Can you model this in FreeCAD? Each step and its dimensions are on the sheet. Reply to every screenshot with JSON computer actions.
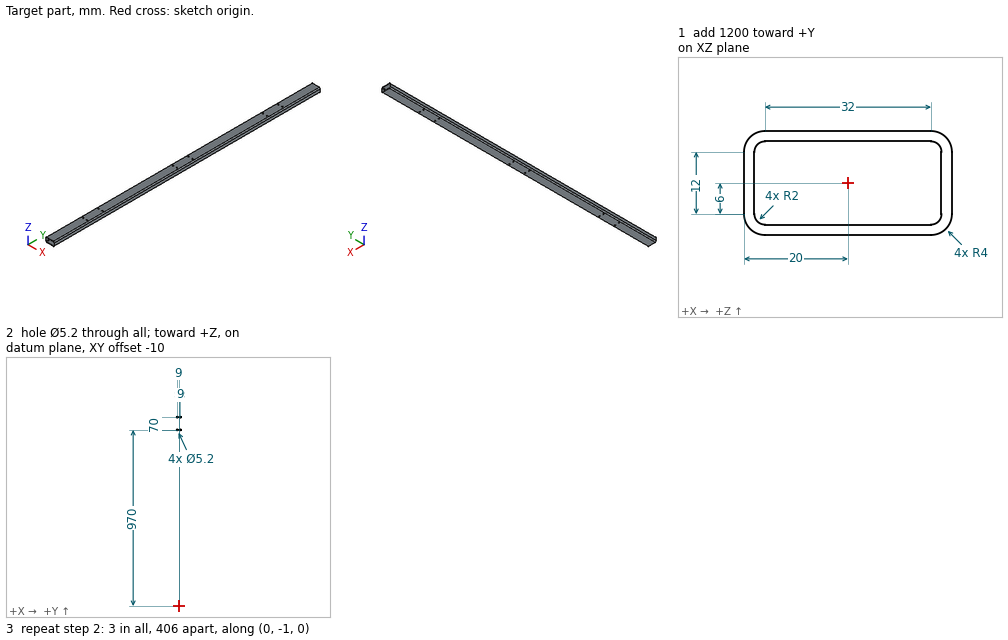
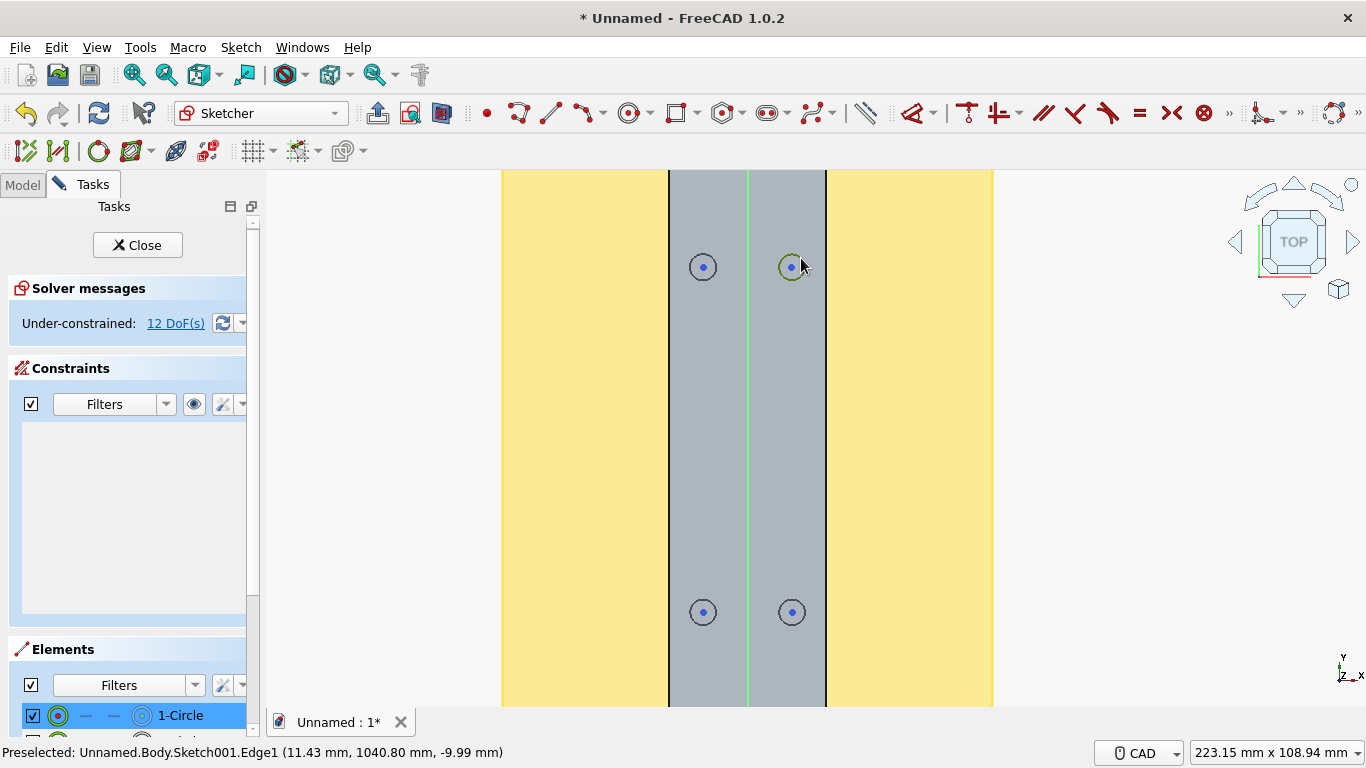
{"action": "left_click", "coordinate": [712, 258]}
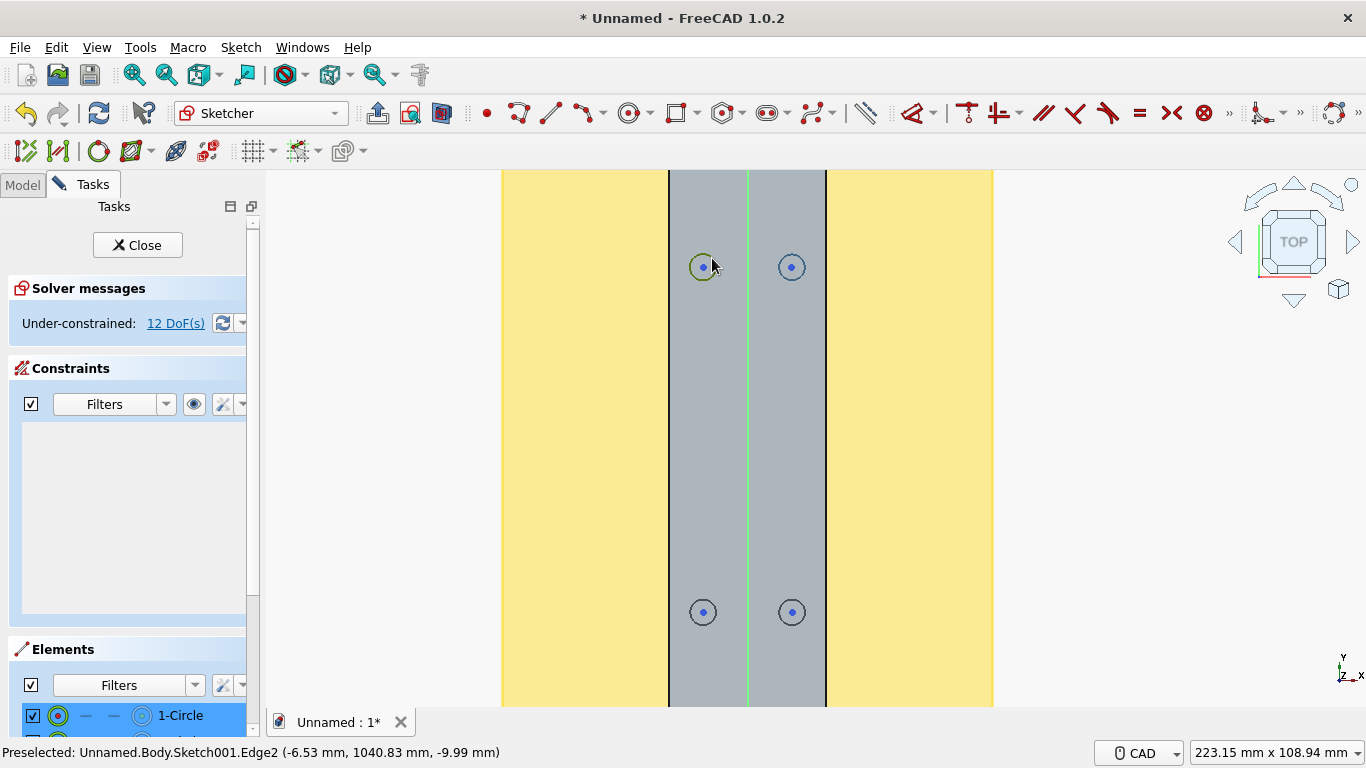
{"action": "left_click", "coordinate": [712, 603]}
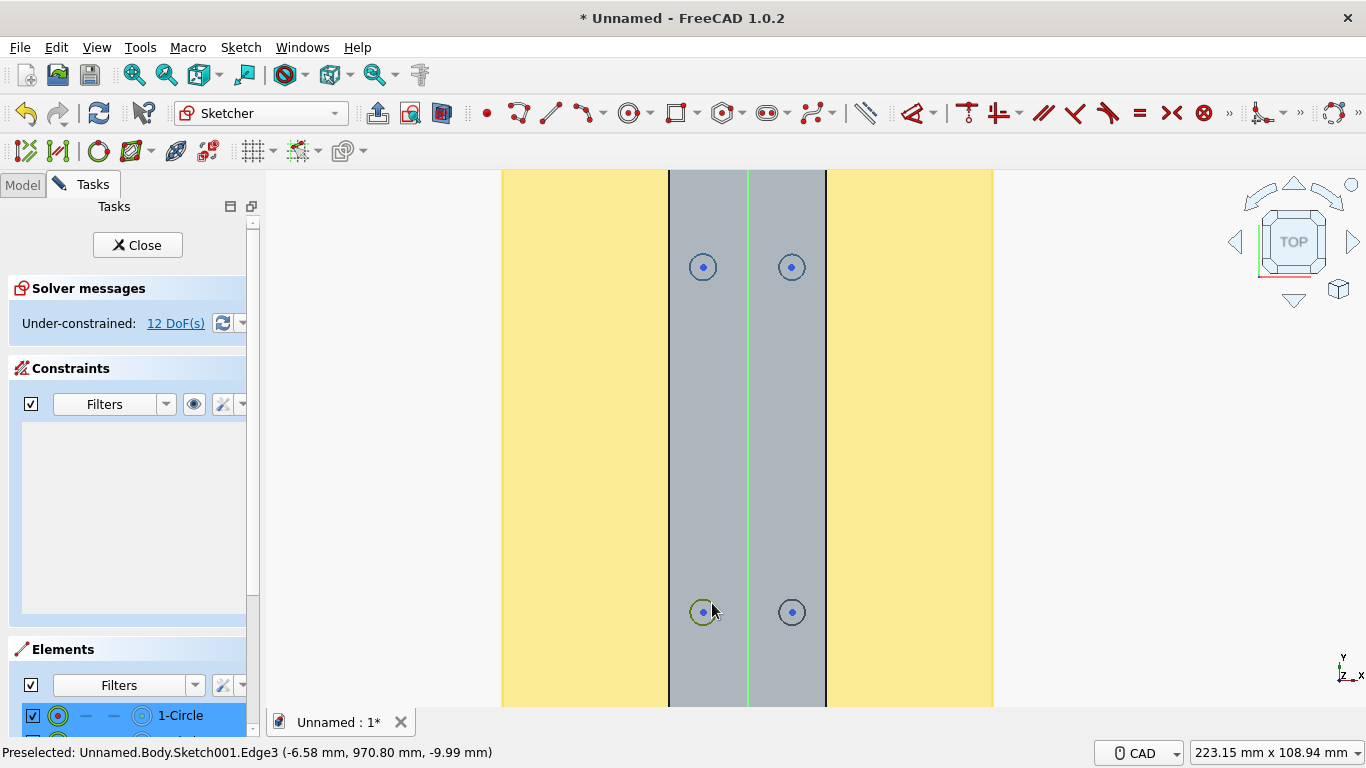
{"action": "left_click", "coordinate": [801, 603]}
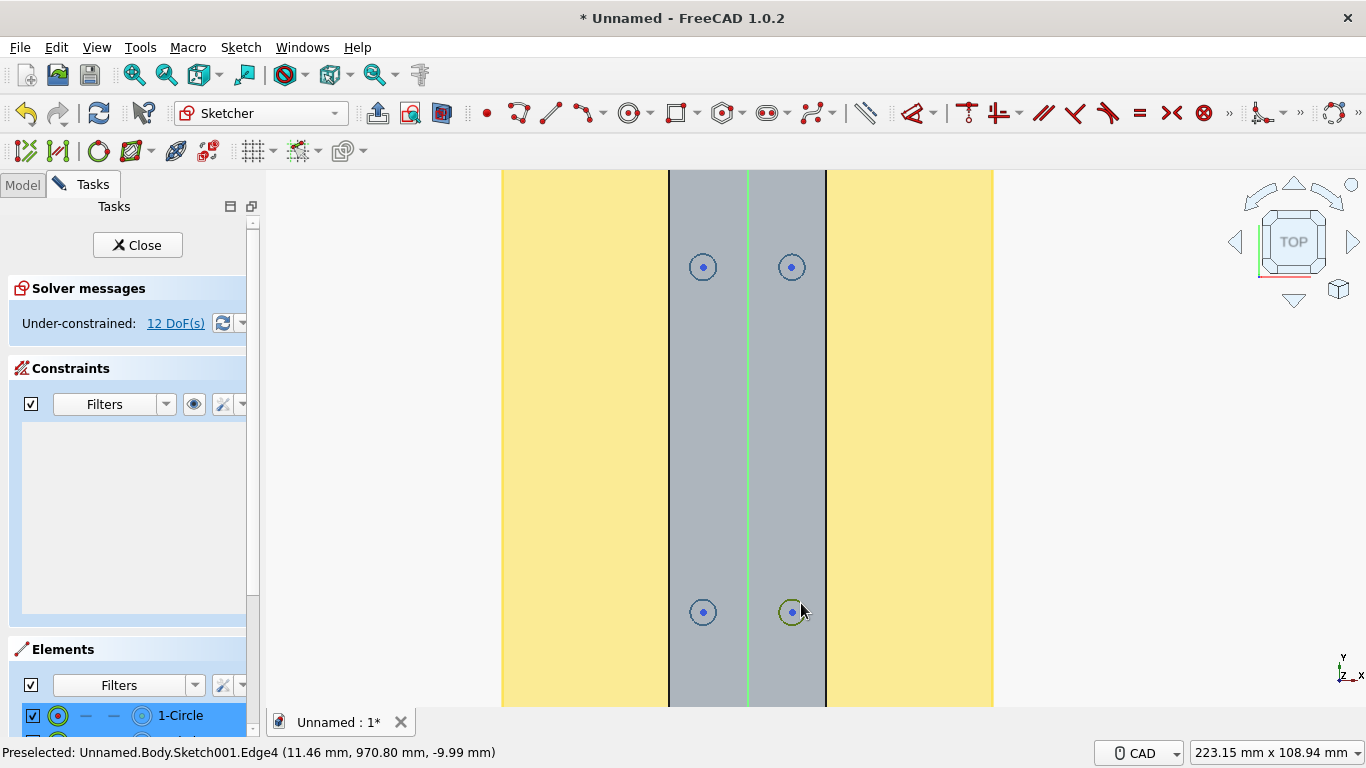
{"action": "left_click", "coordinate": [1140, 114]}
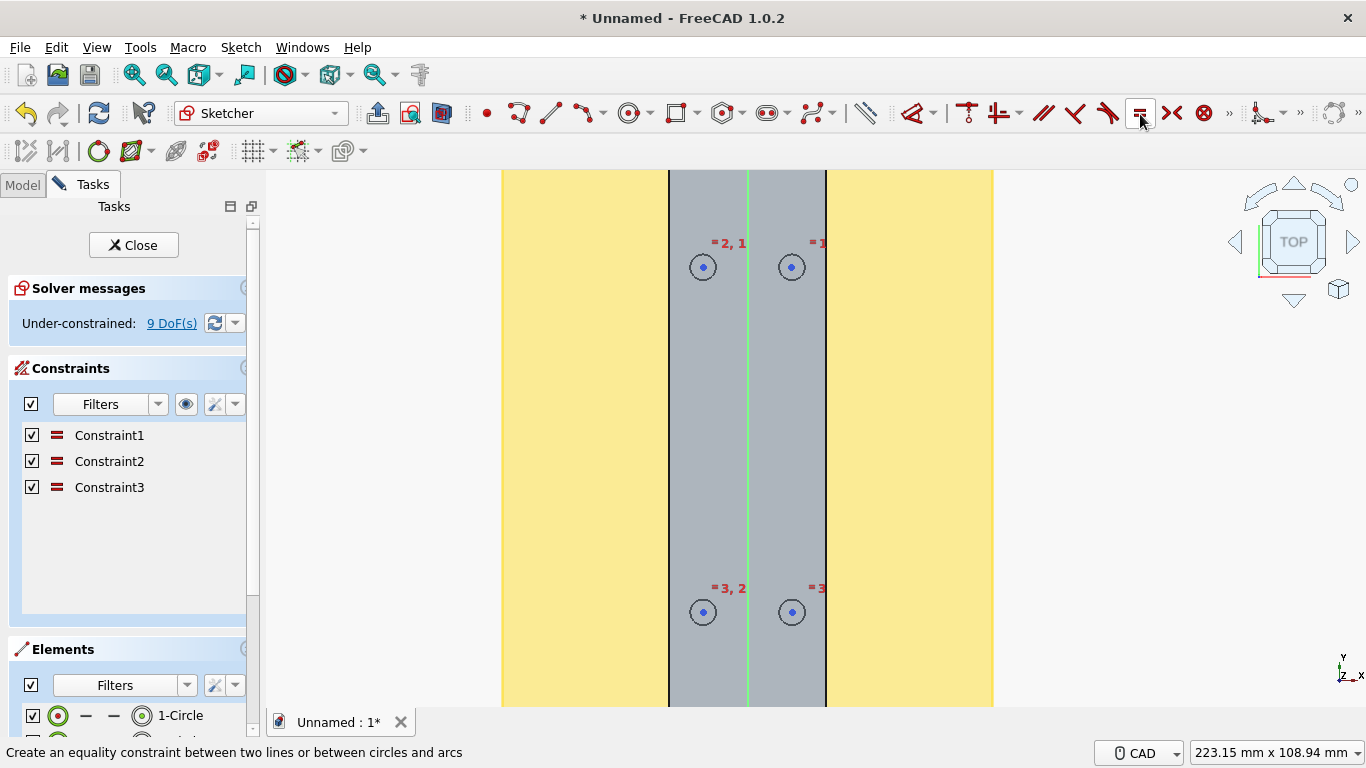
{"action": "left_click", "coordinate": [792, 267]}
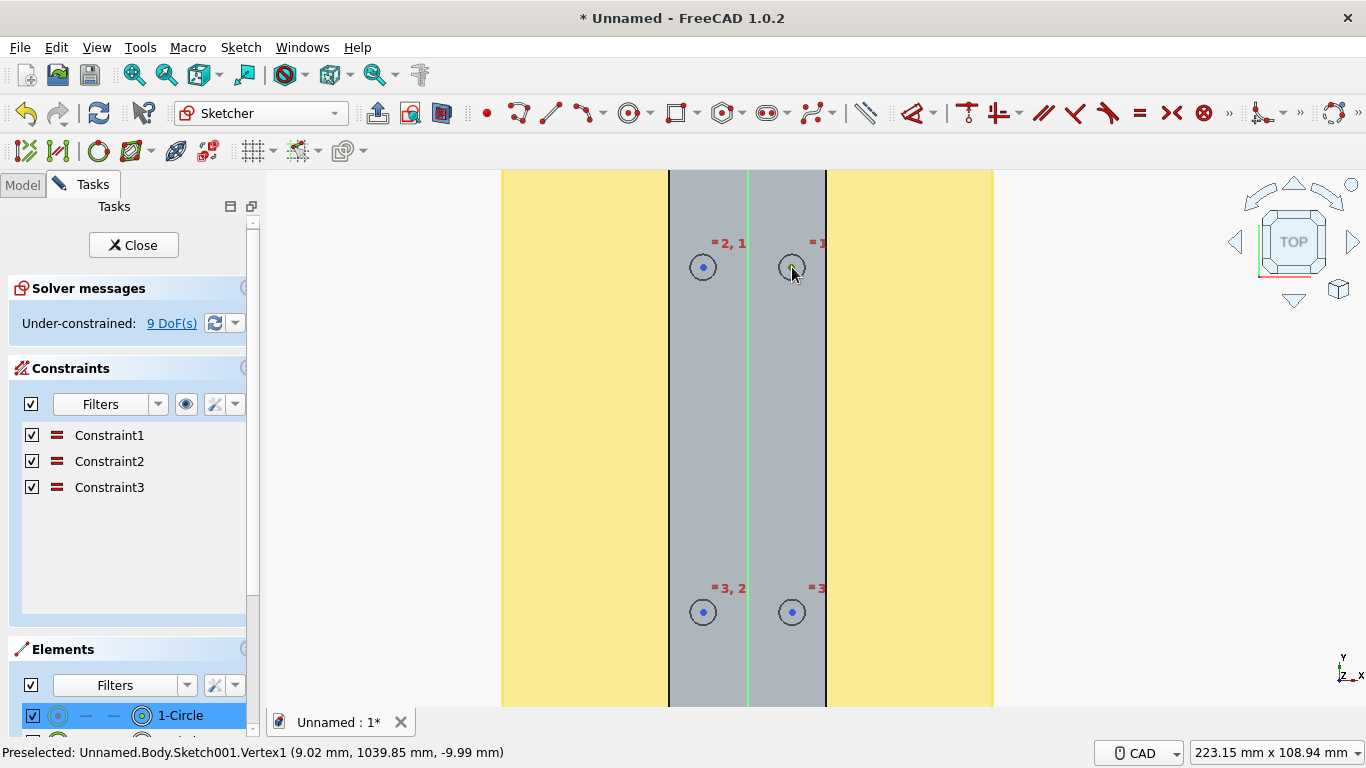
{"action": "left_click", "coordinate": [703, 267]}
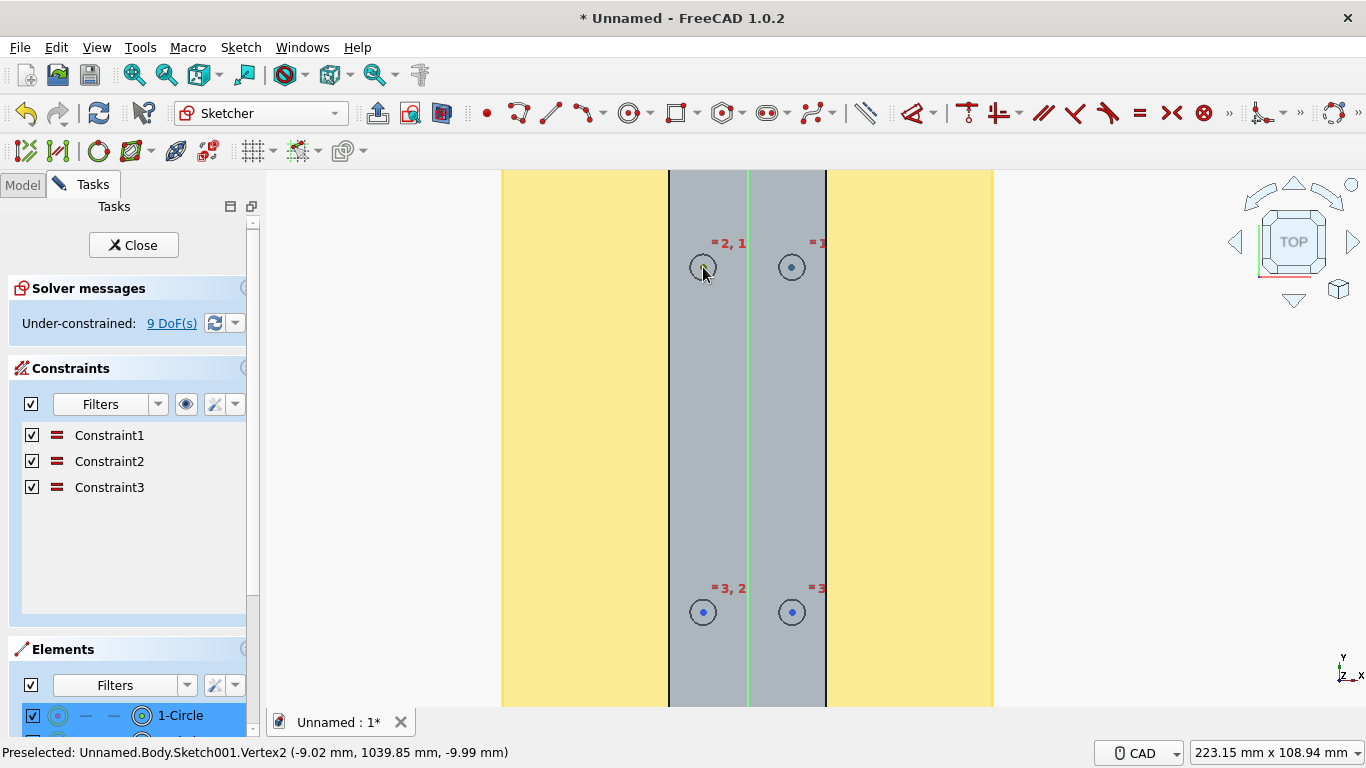
{"action": "left_click", "coordinate": [1022, 114]}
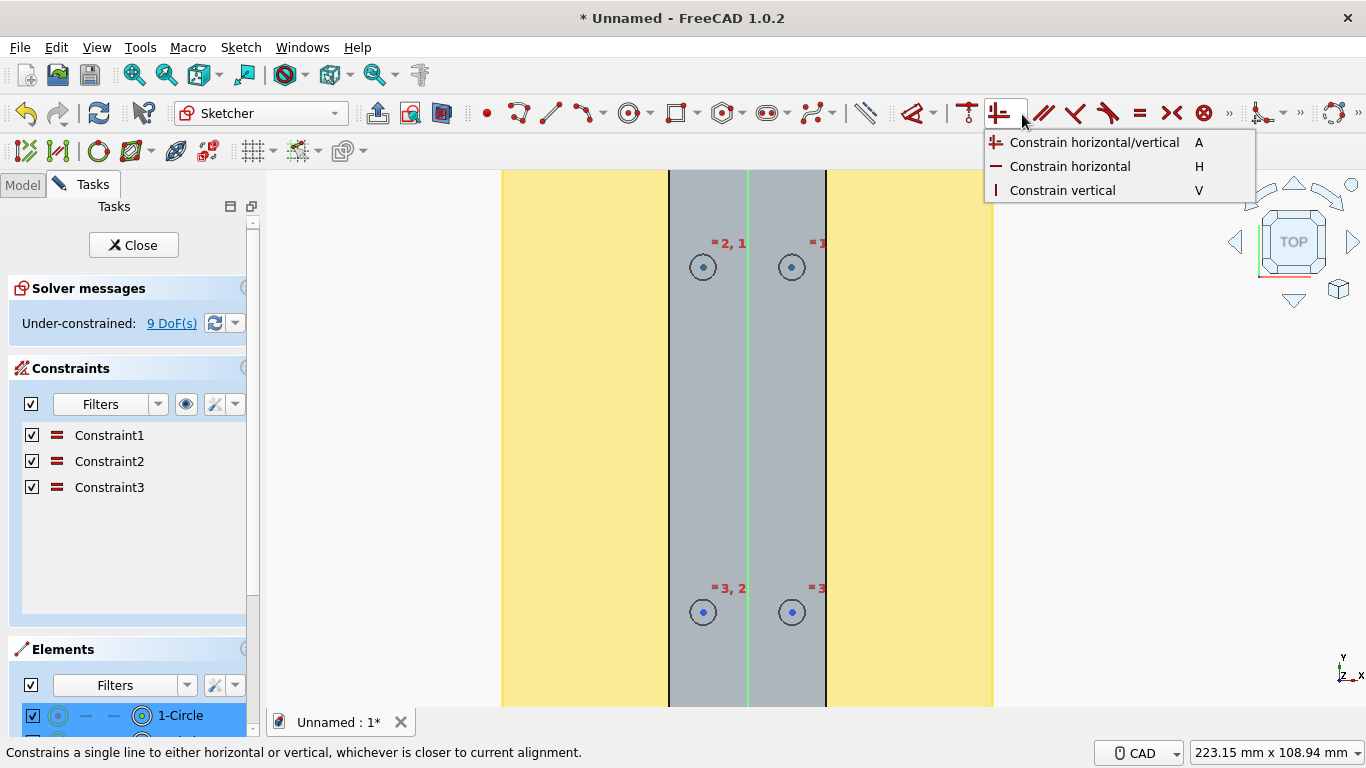
{"action": "left_click", "coordinate": [1120, 166]}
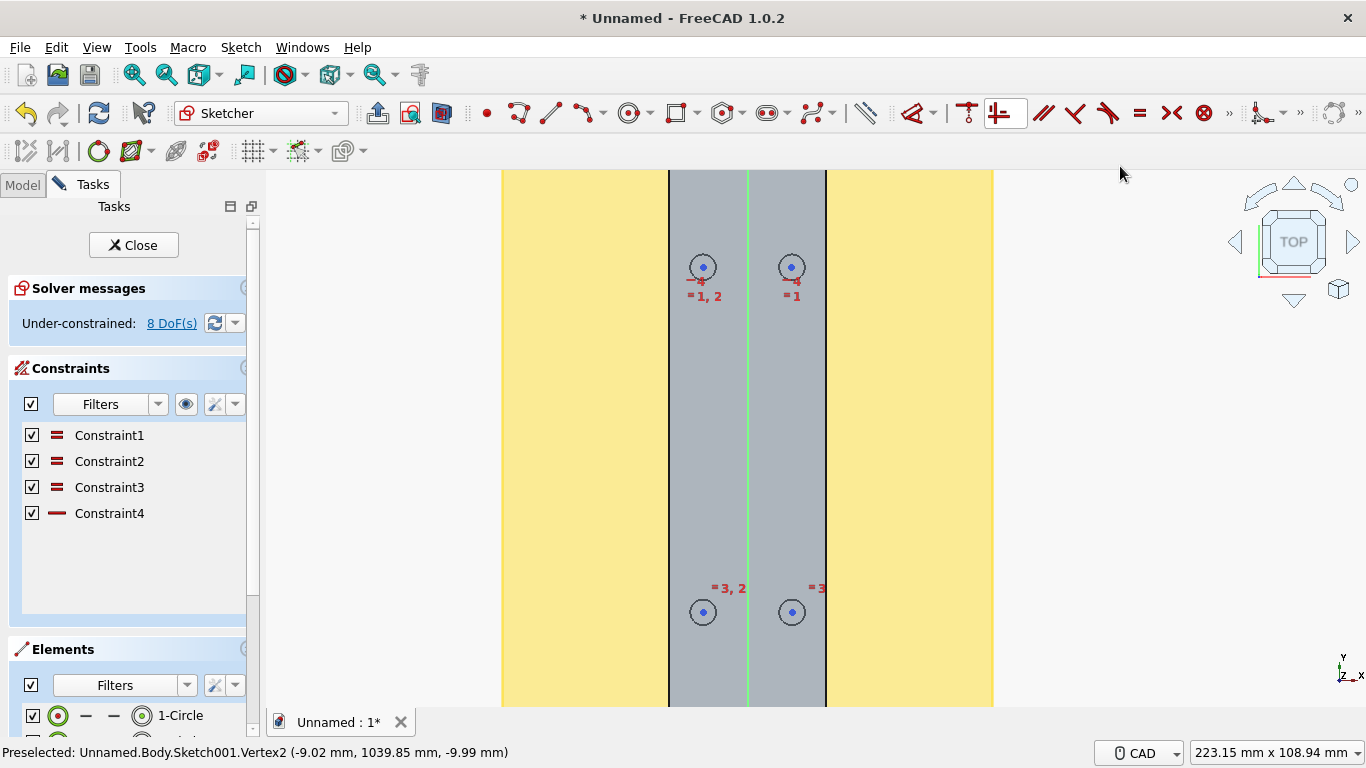
{"action": "left_click", "coordinate": [703, 267]}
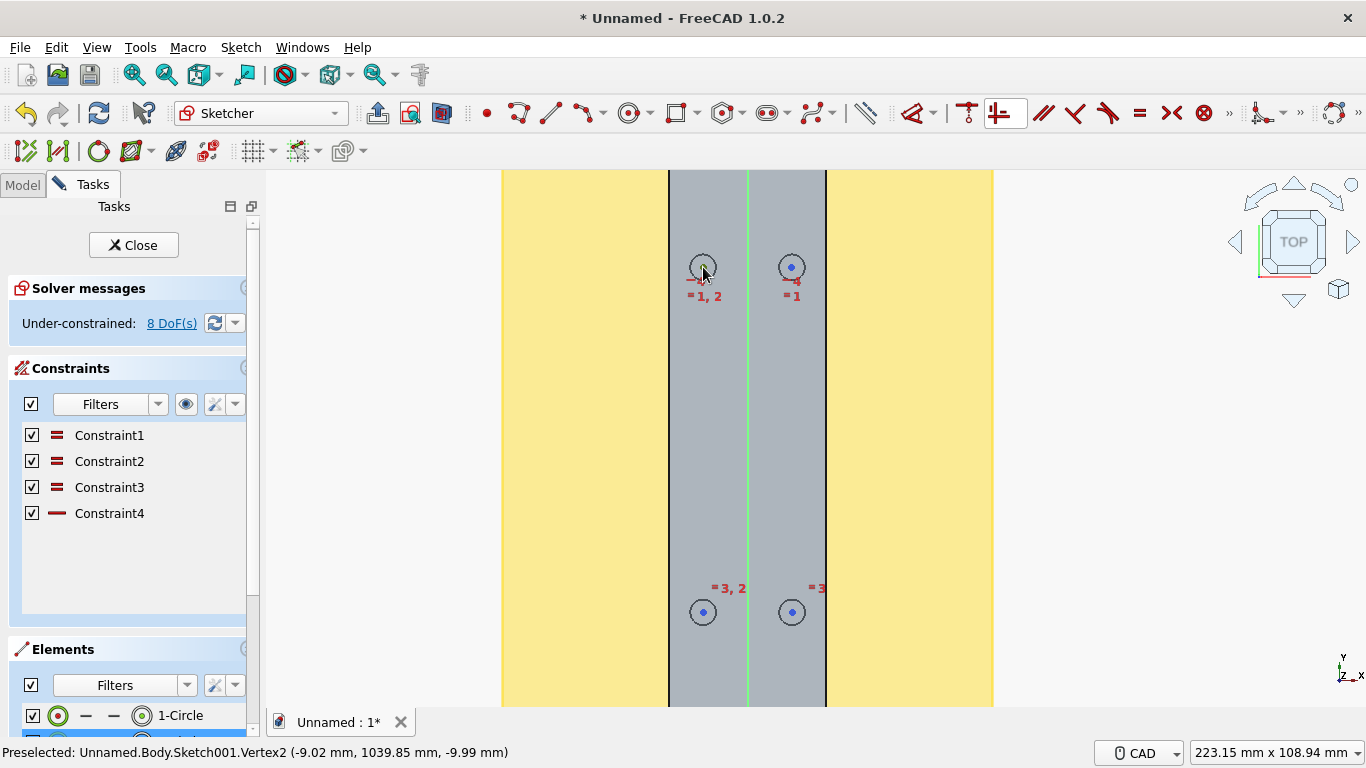
{"action": "left_click", "coordinate": [703, 612]}